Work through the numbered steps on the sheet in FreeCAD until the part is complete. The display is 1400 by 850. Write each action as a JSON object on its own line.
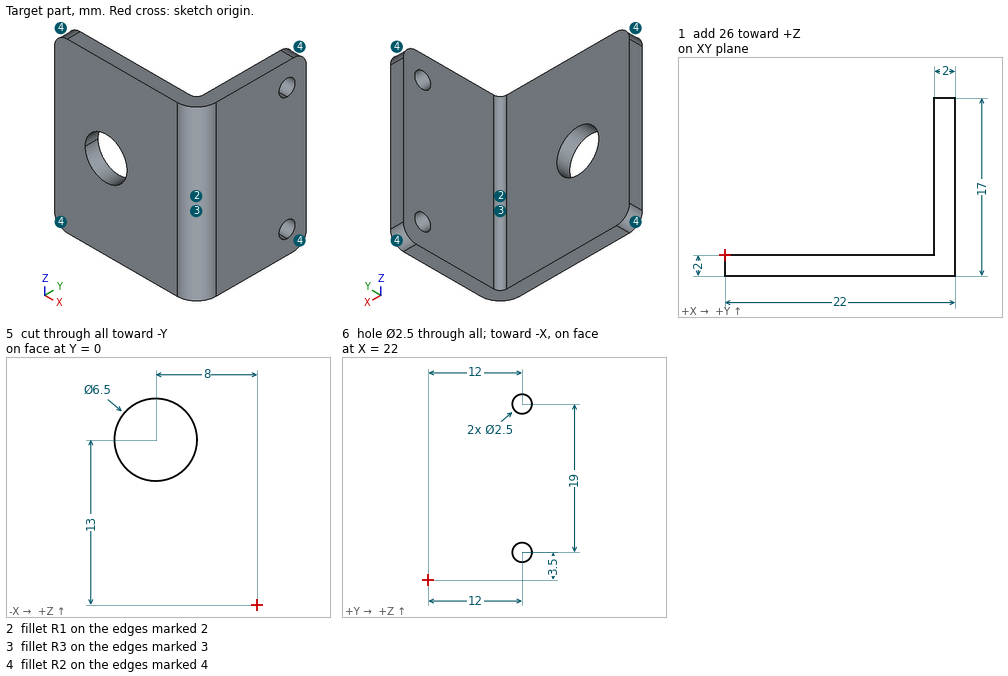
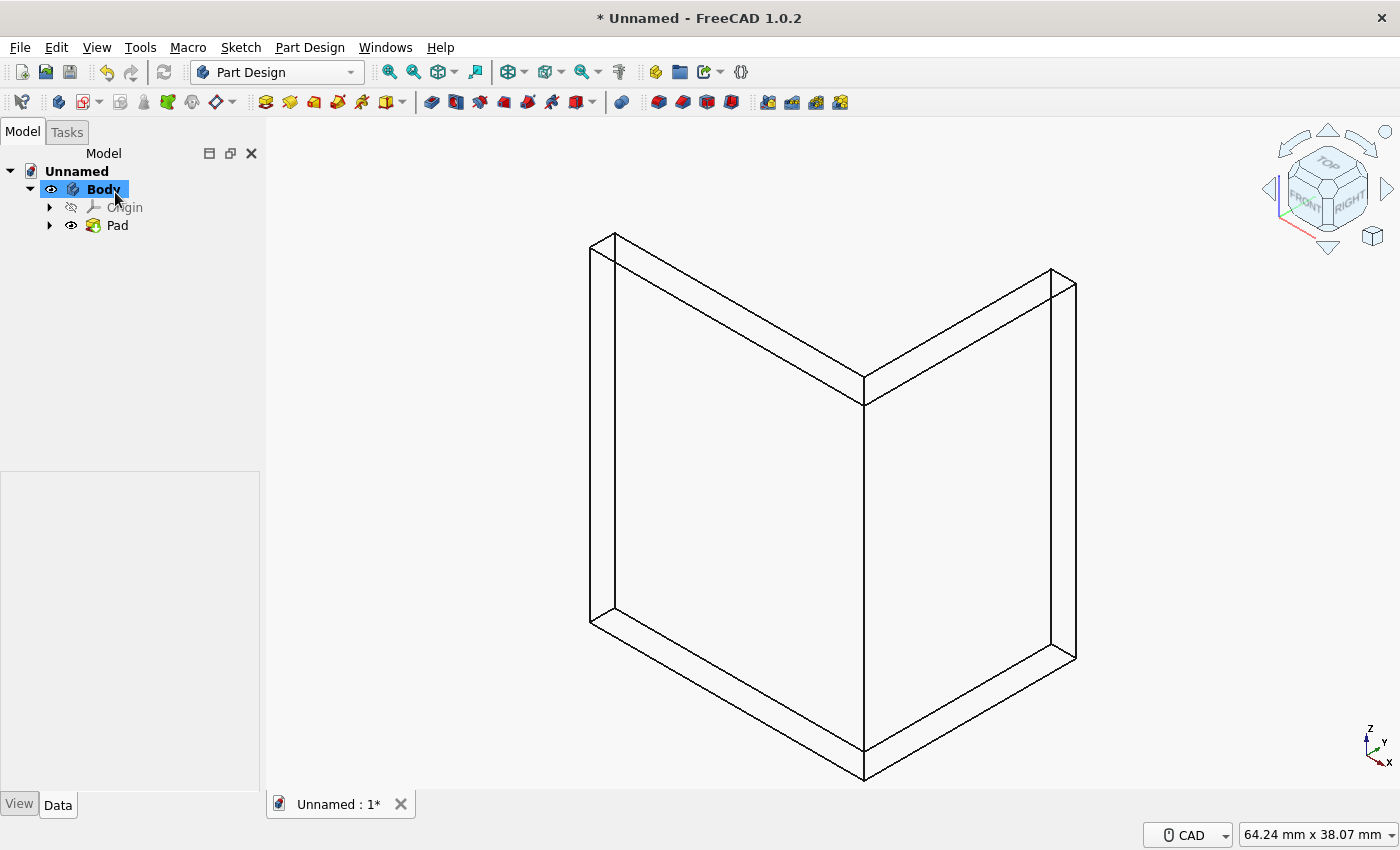
{"action": "key", "text": "2"}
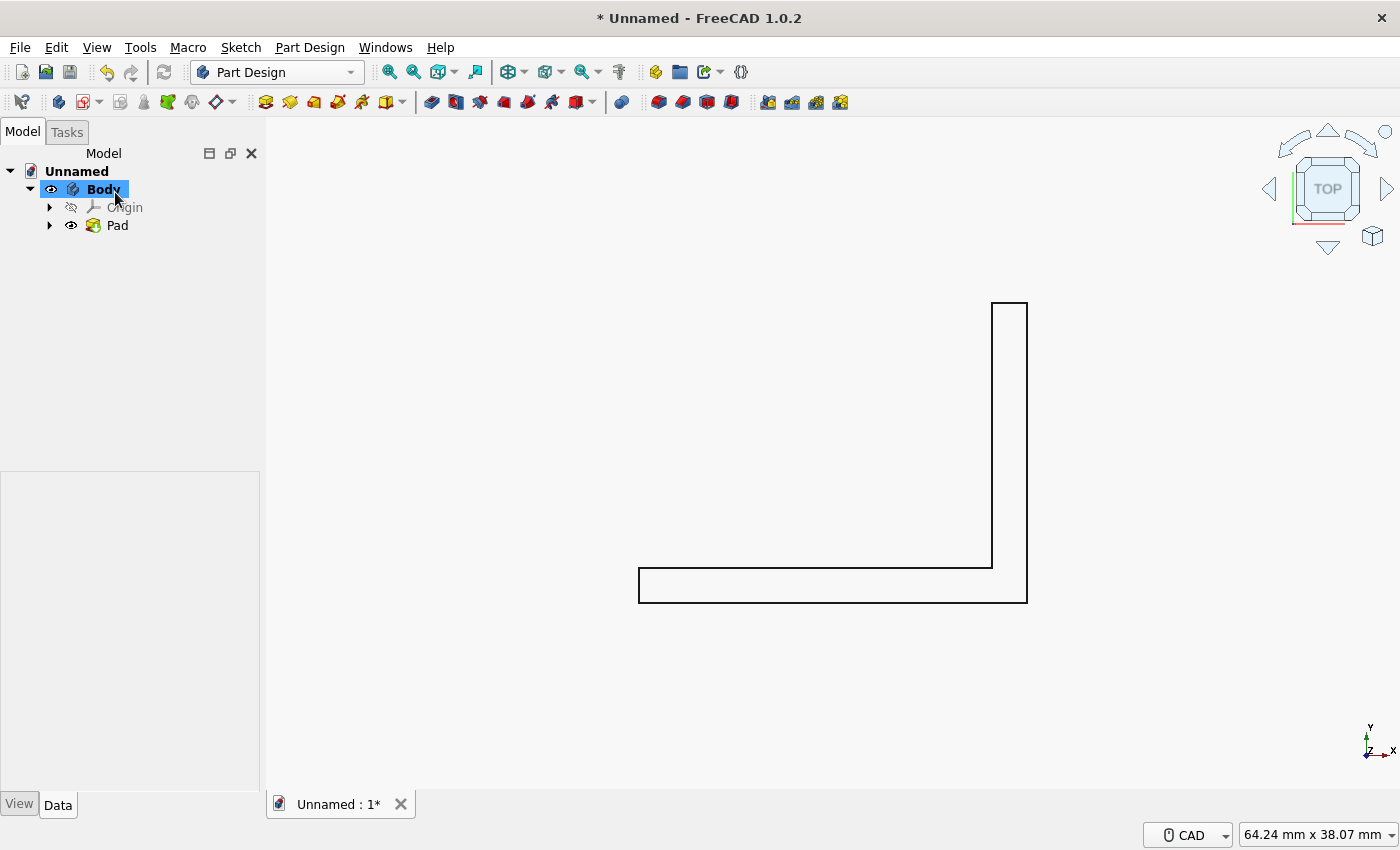
{"action": "left_click", "coordinate": [390, 72]}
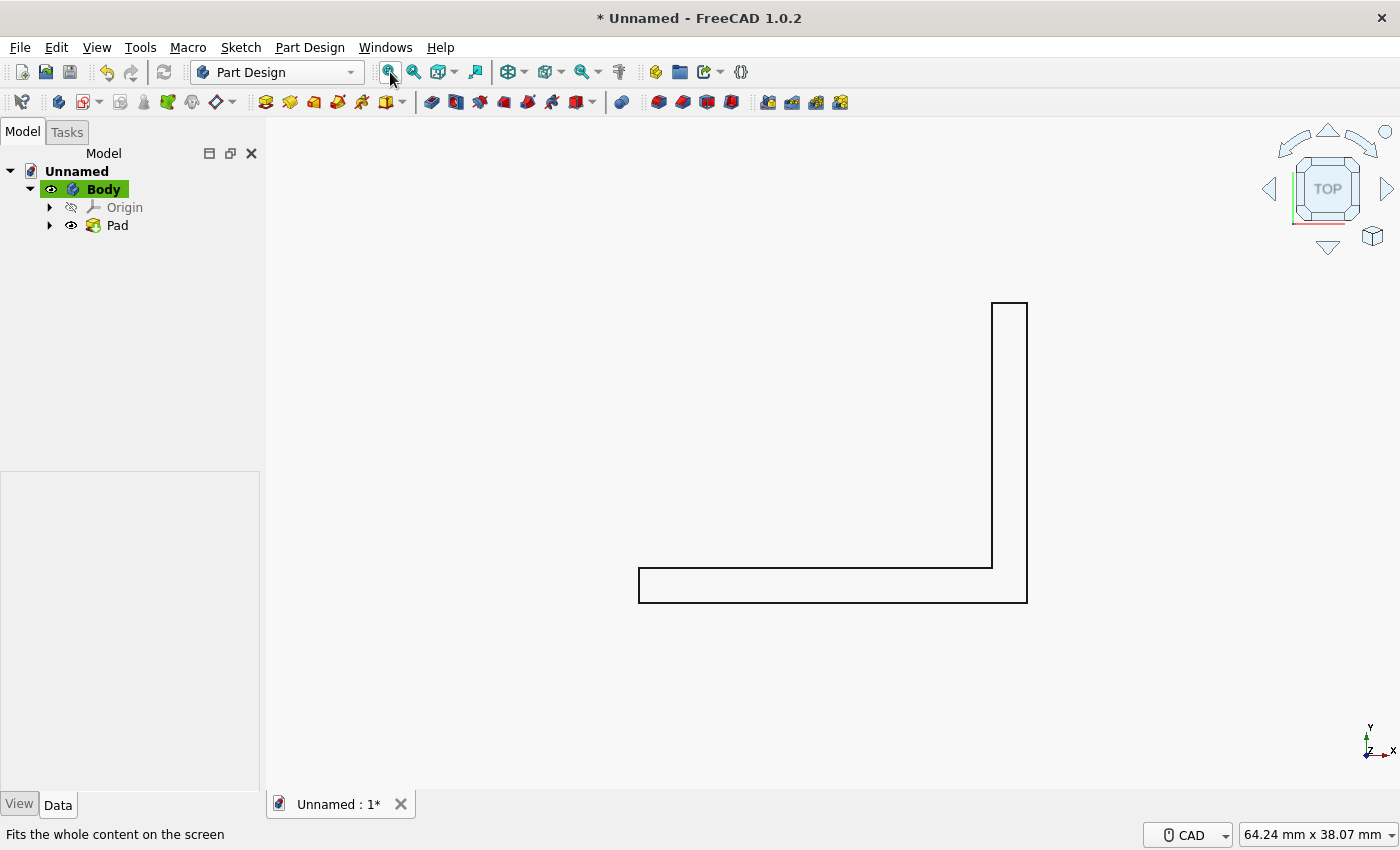
{"action": "key", "text": "1"}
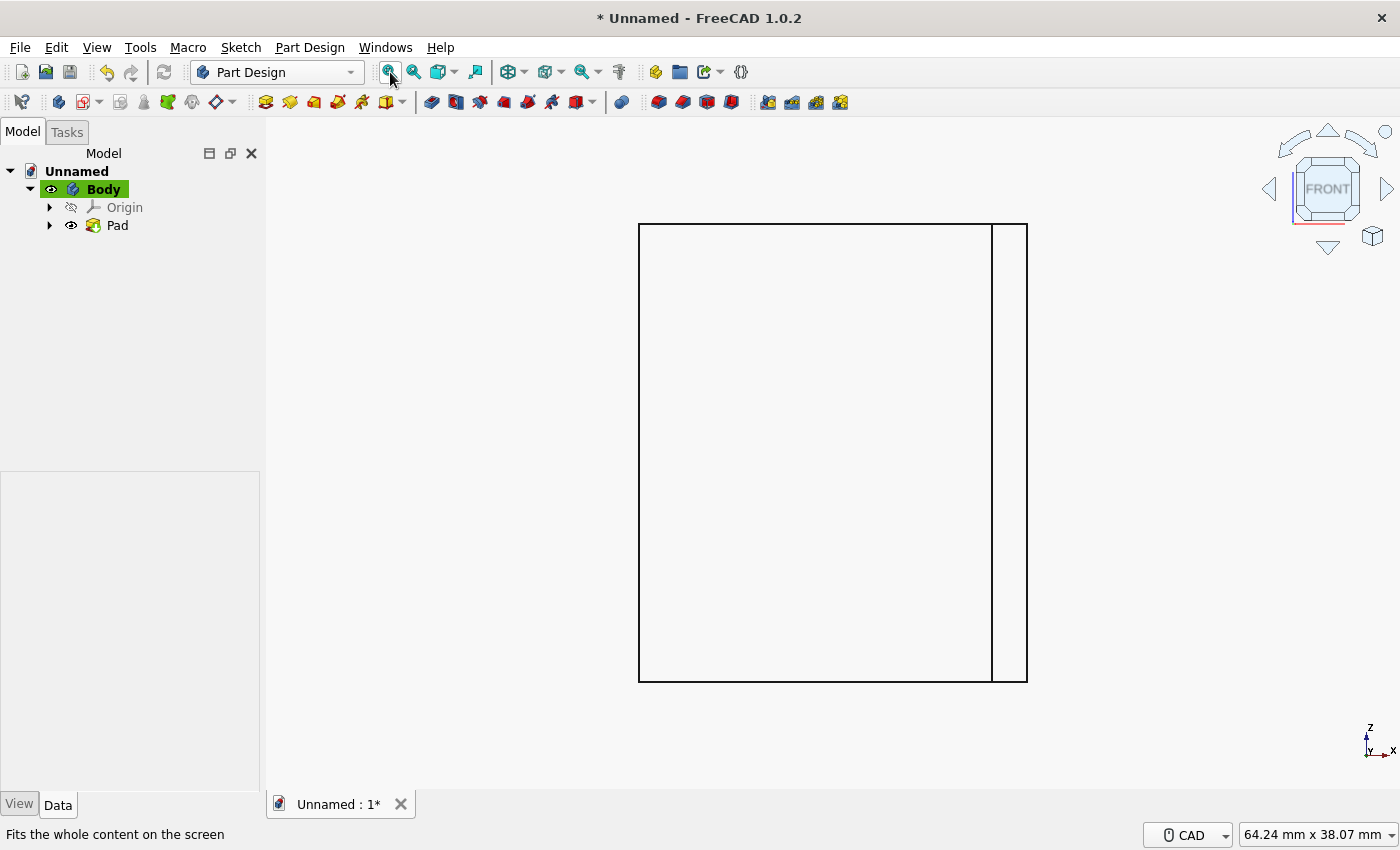
{"action": "left_click", "coordinate": [992, 452]}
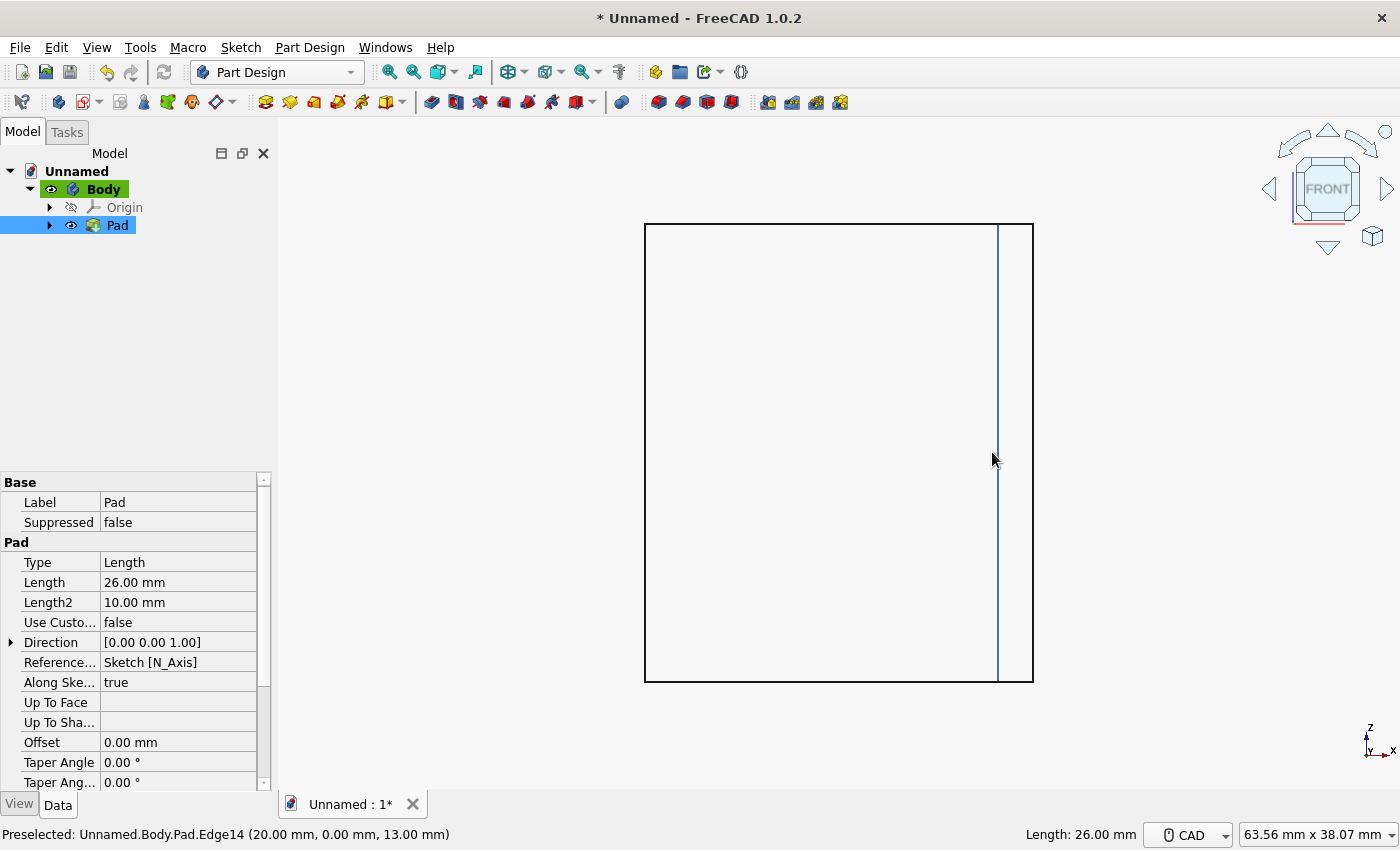
{"action": "key", "text": "v 1"}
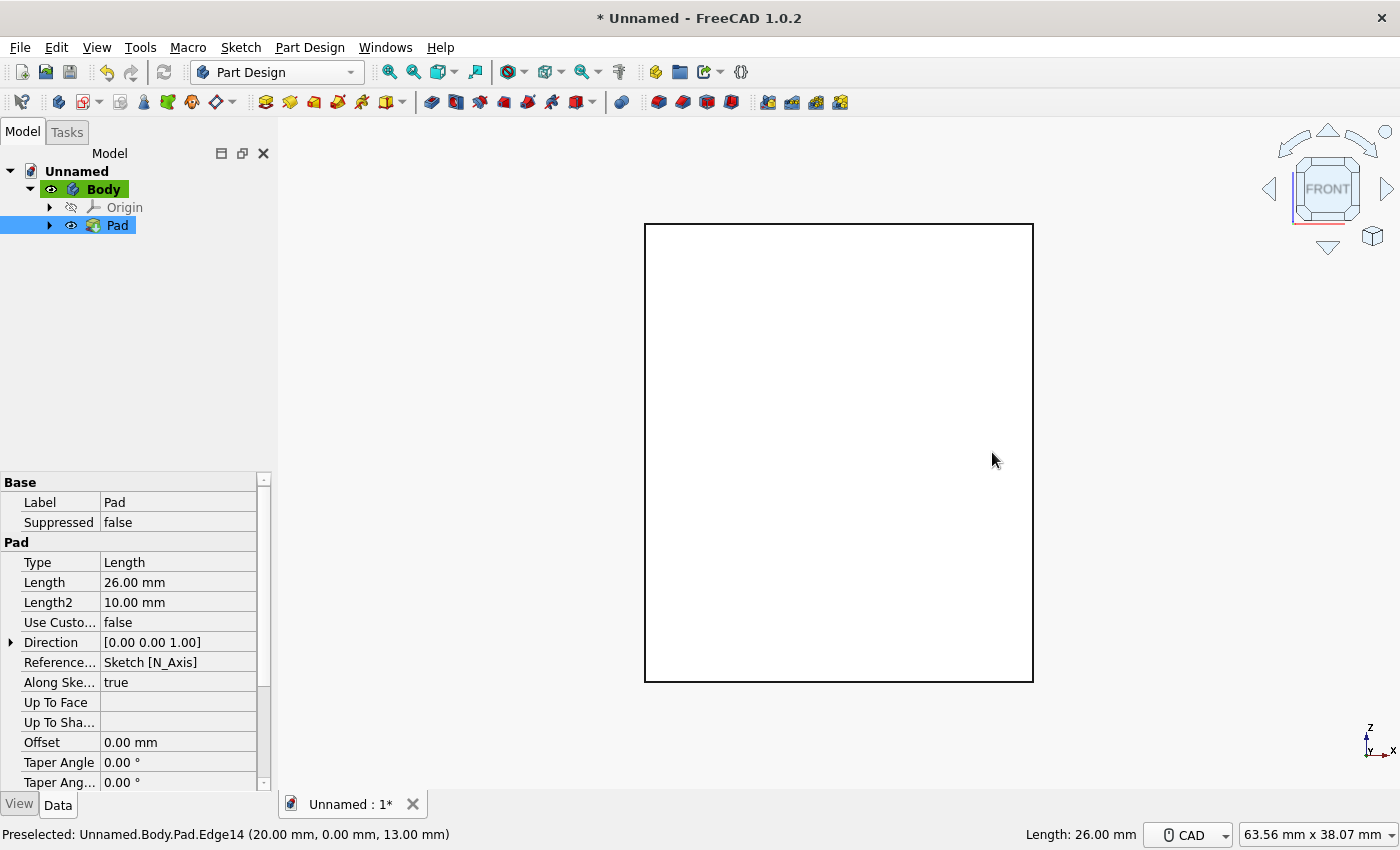
{"action": "left_click", "coordinate": [660, 102]}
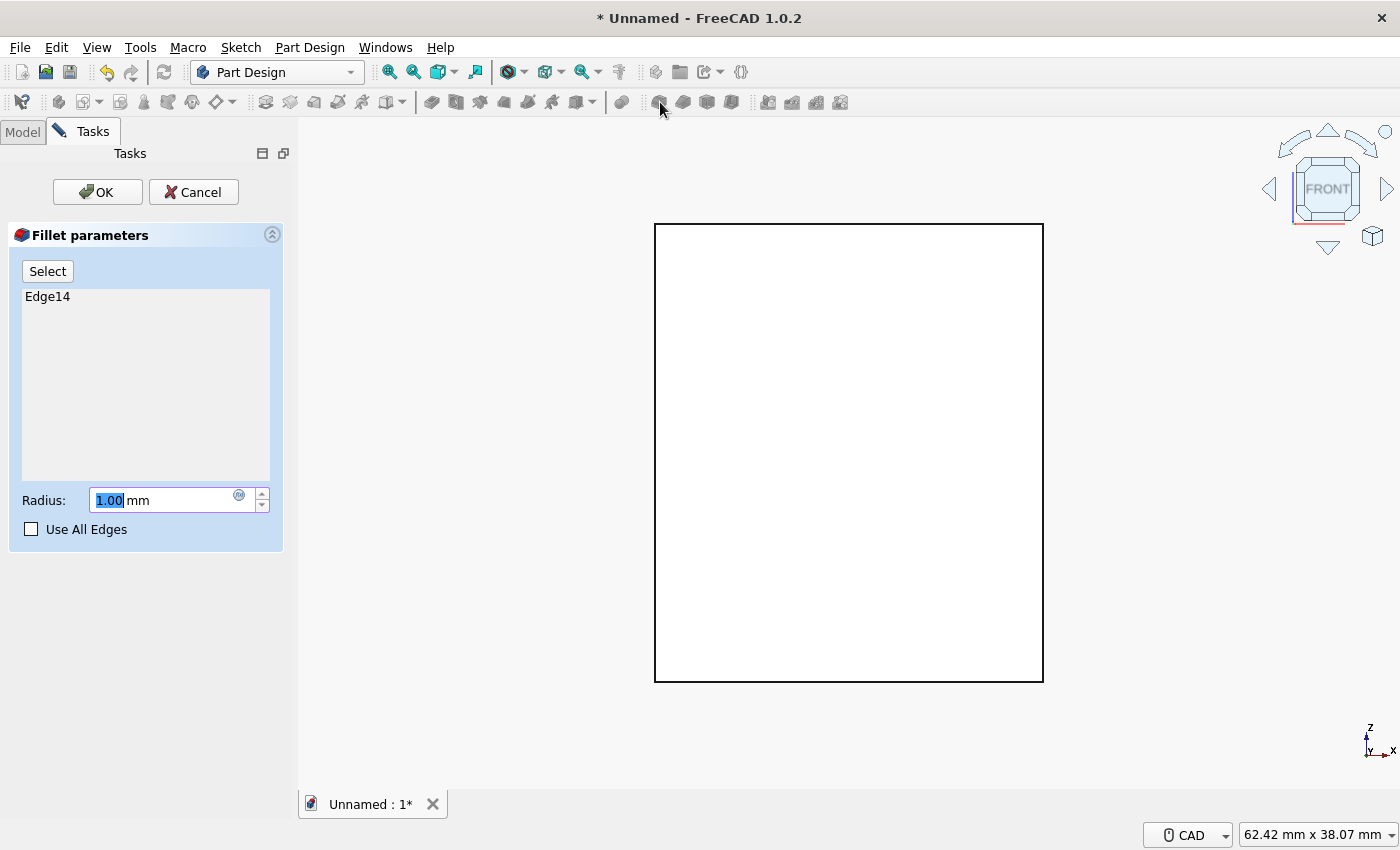
{"action": "type", "text": "1"}
{"action": "key", "text": "Tab"}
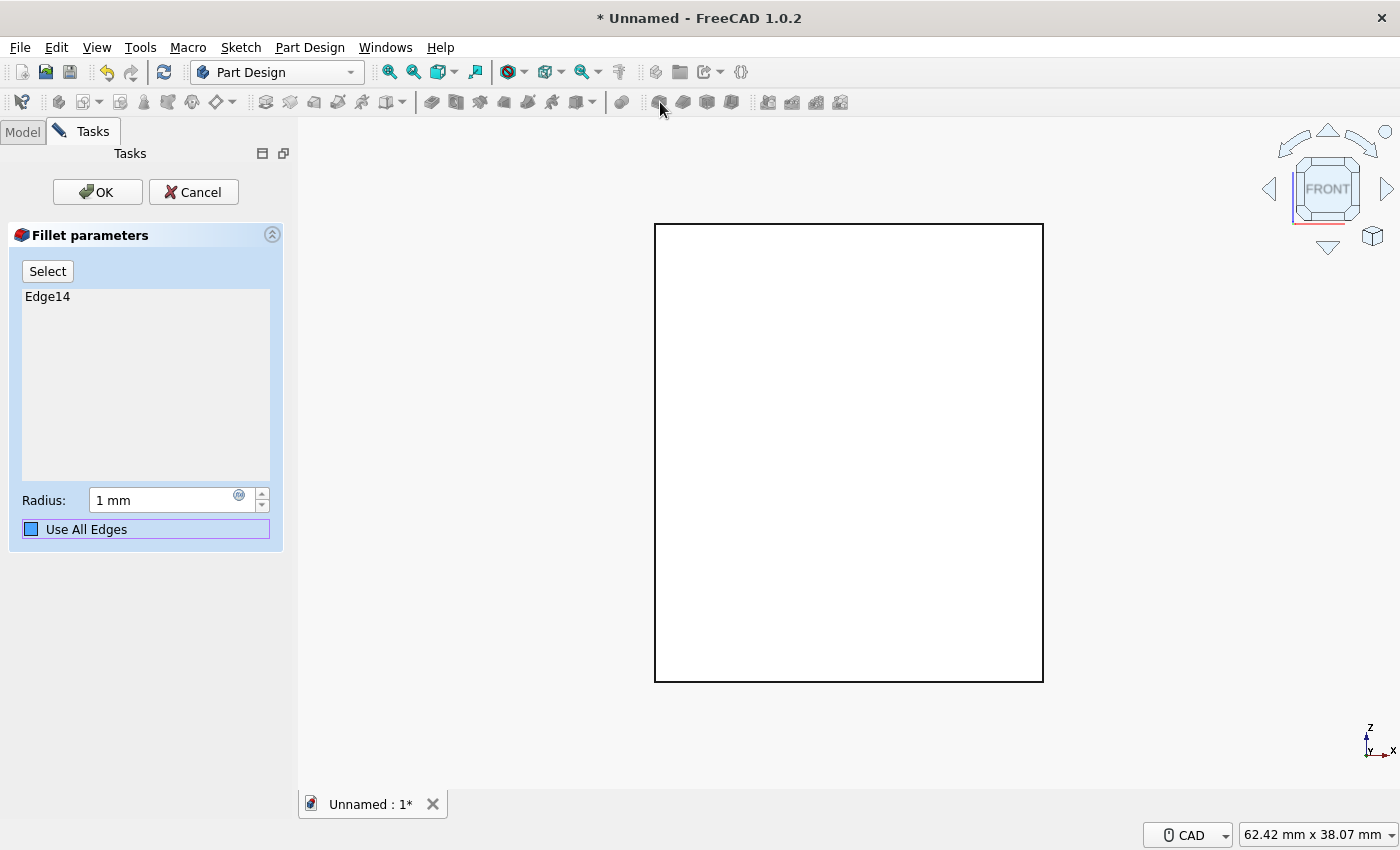
{"action": "left_click", "coordinate": [98, 192]}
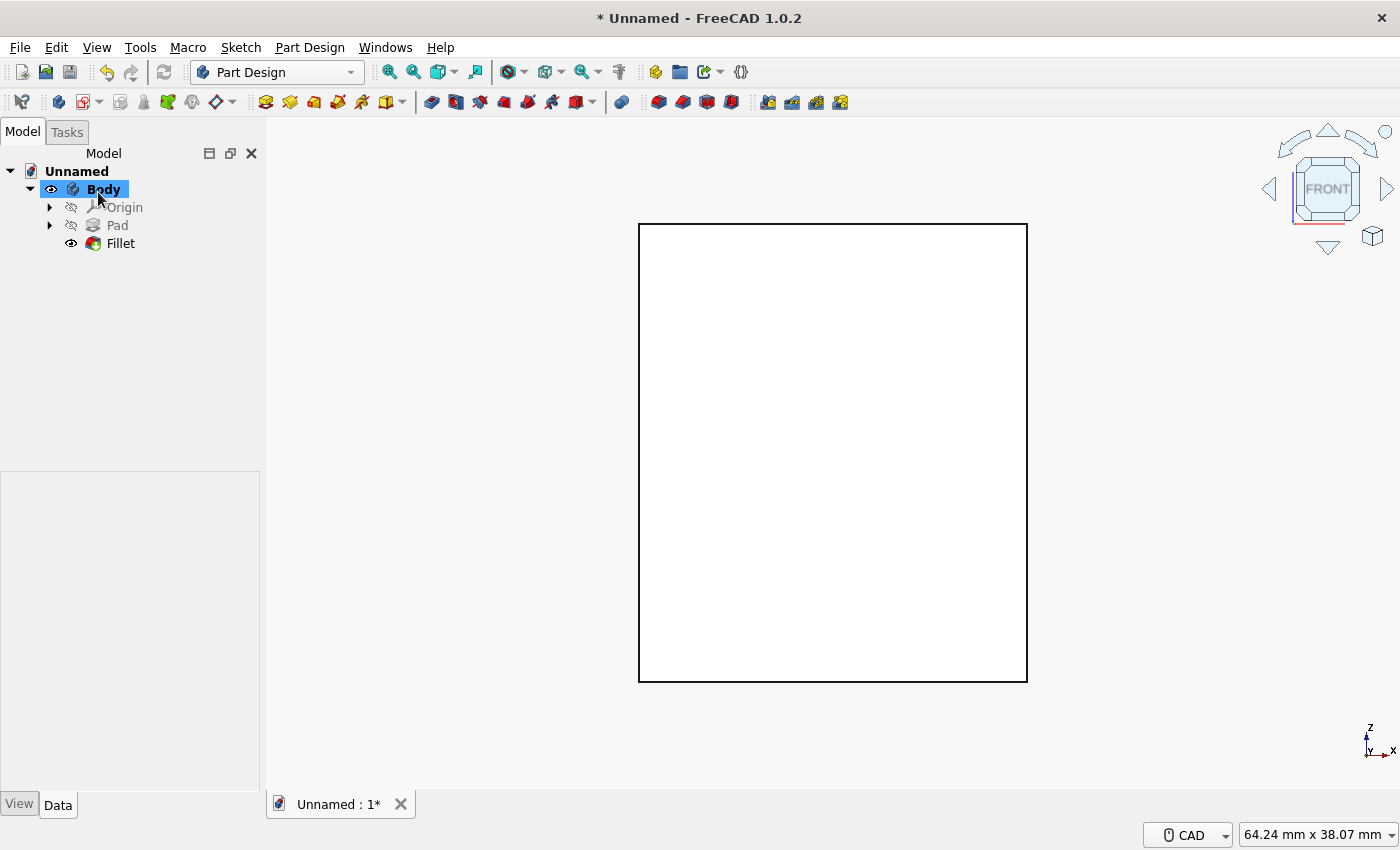
{"action": "left_click", "coordinate": [1027, 452]}